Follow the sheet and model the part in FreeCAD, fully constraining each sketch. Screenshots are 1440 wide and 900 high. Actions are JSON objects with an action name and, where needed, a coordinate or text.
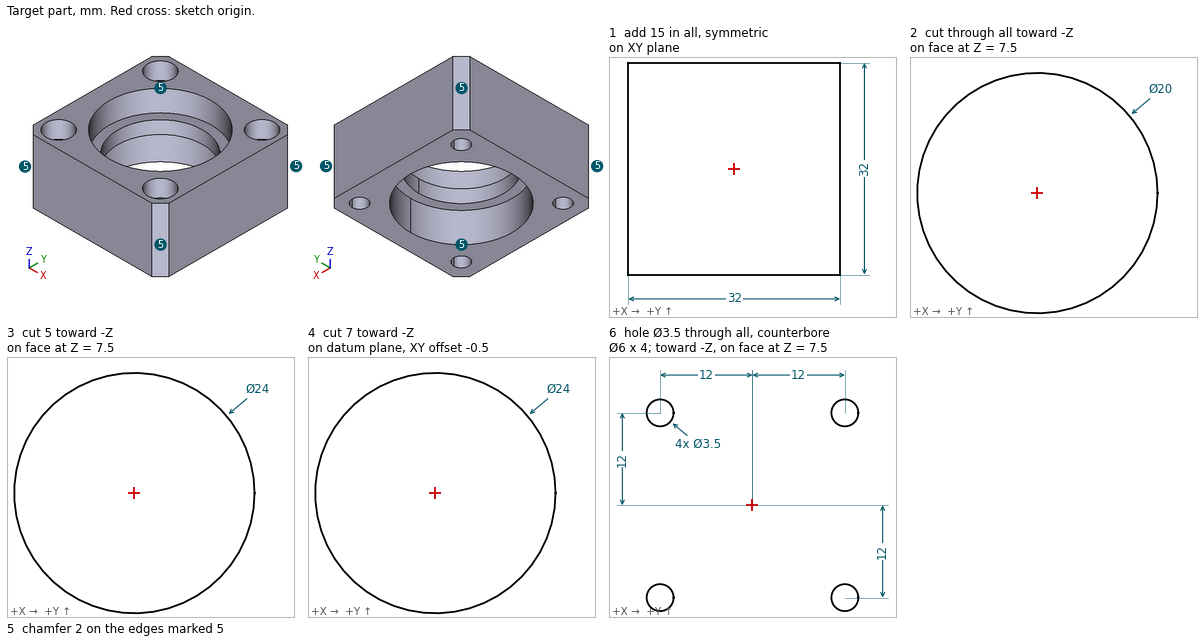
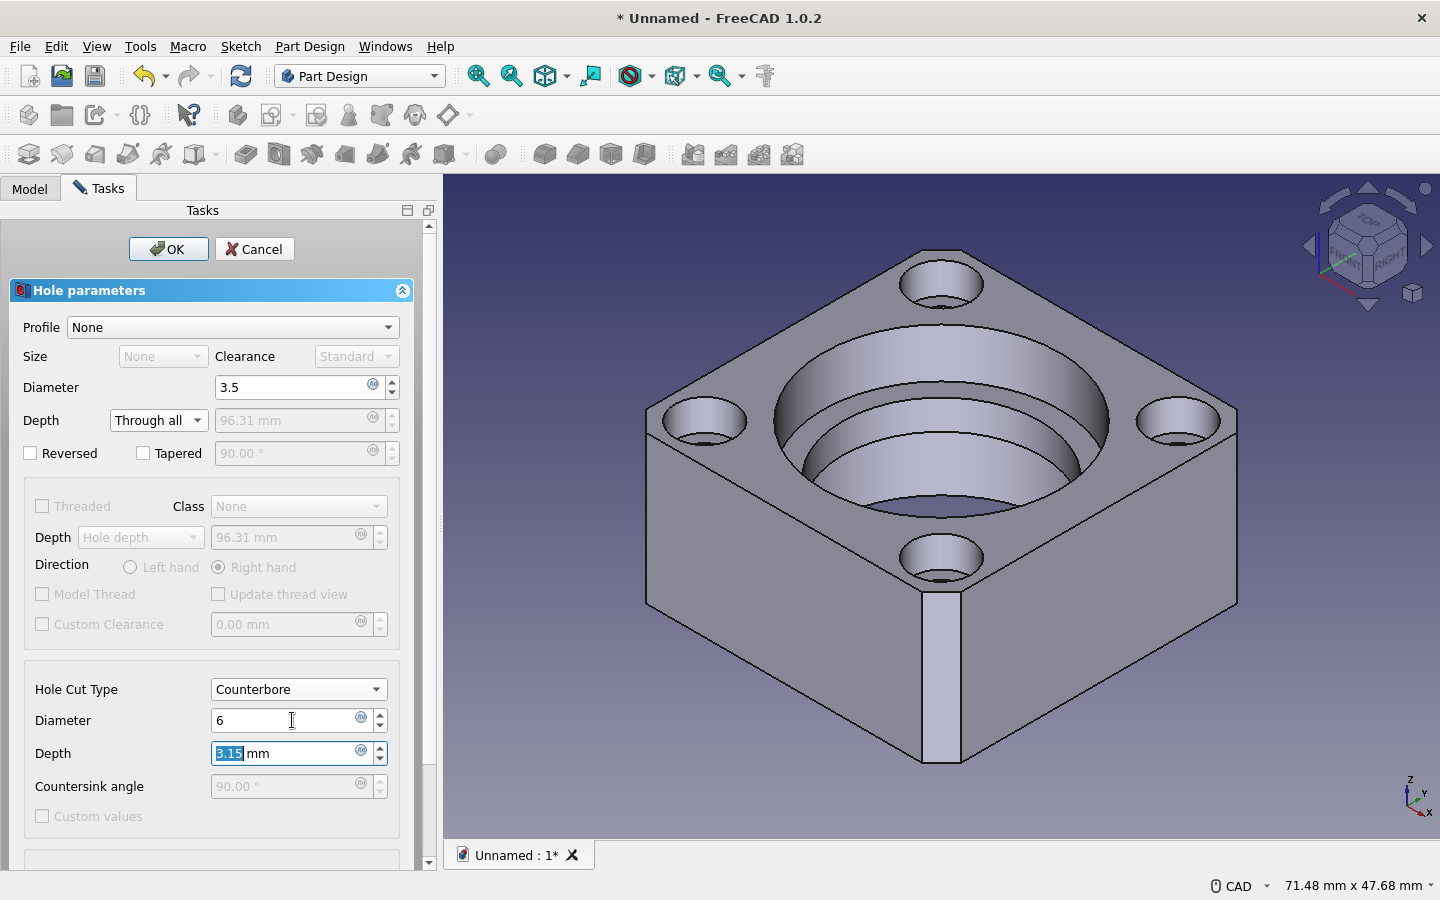
{"action": "type", "text": "4"}
{"action": "key", "text": "Tab"}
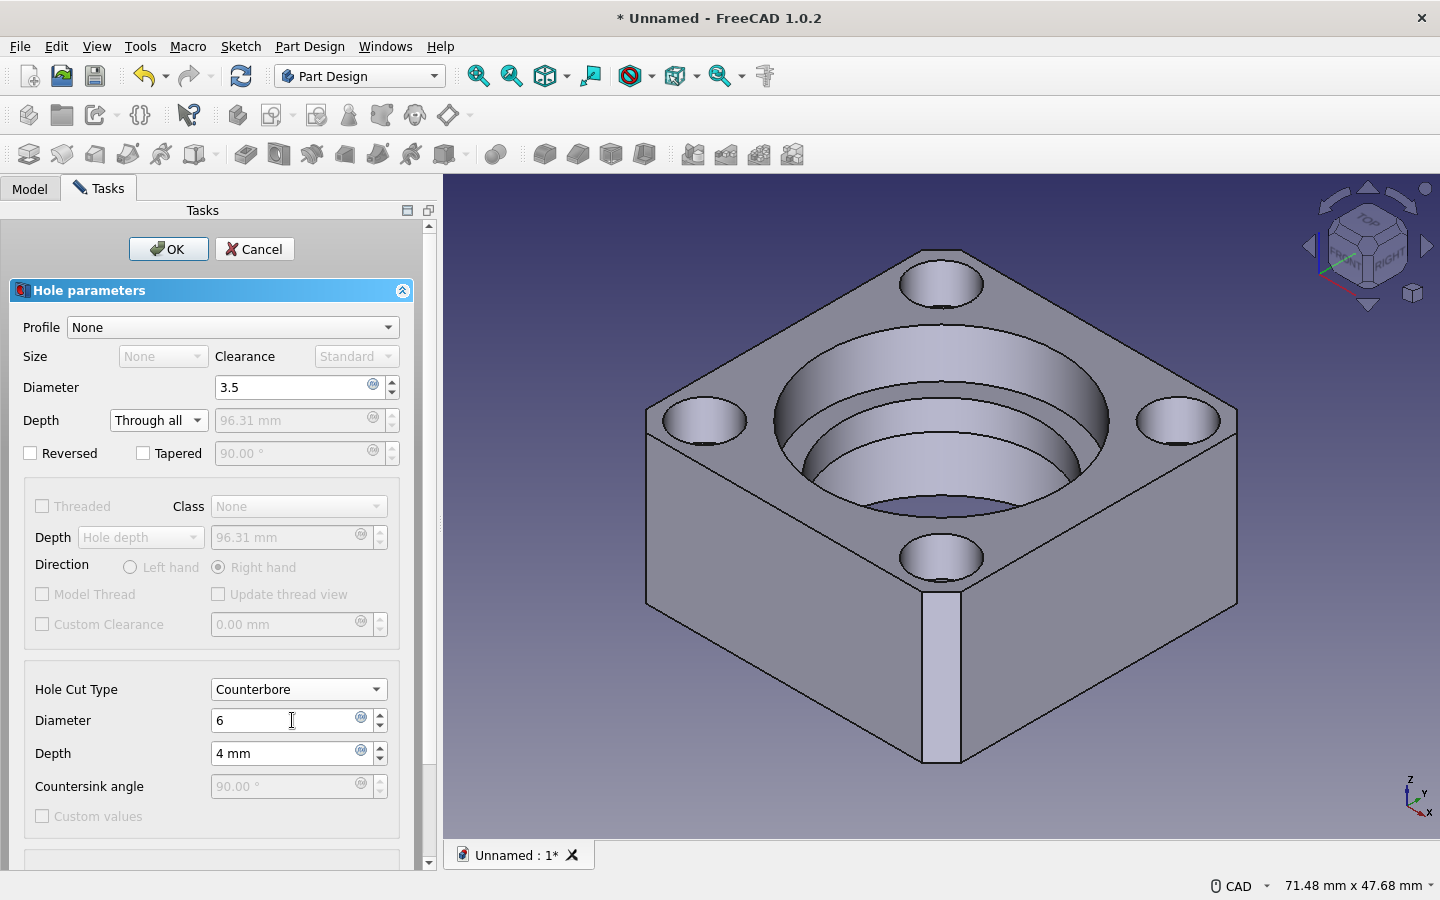
{"action": "left_click", "coordinate": [169, 249]}